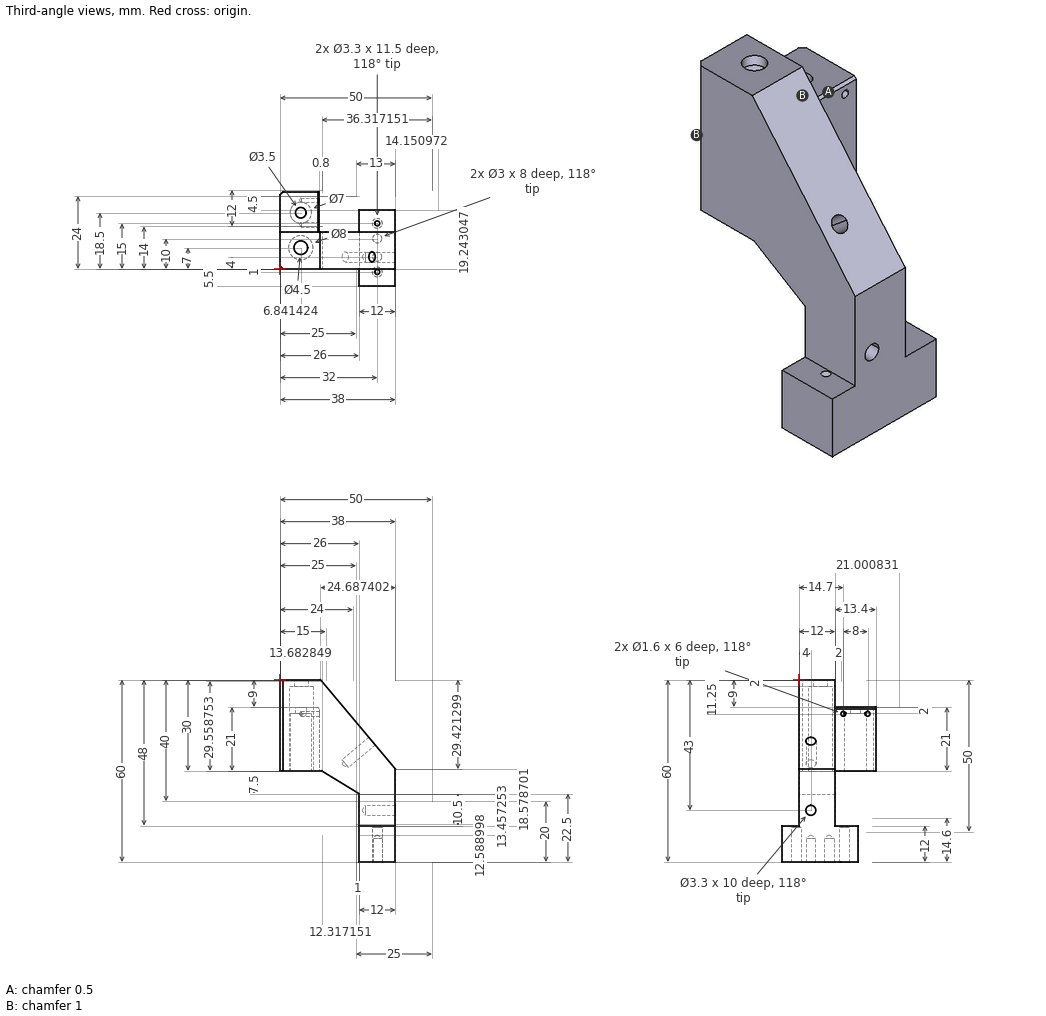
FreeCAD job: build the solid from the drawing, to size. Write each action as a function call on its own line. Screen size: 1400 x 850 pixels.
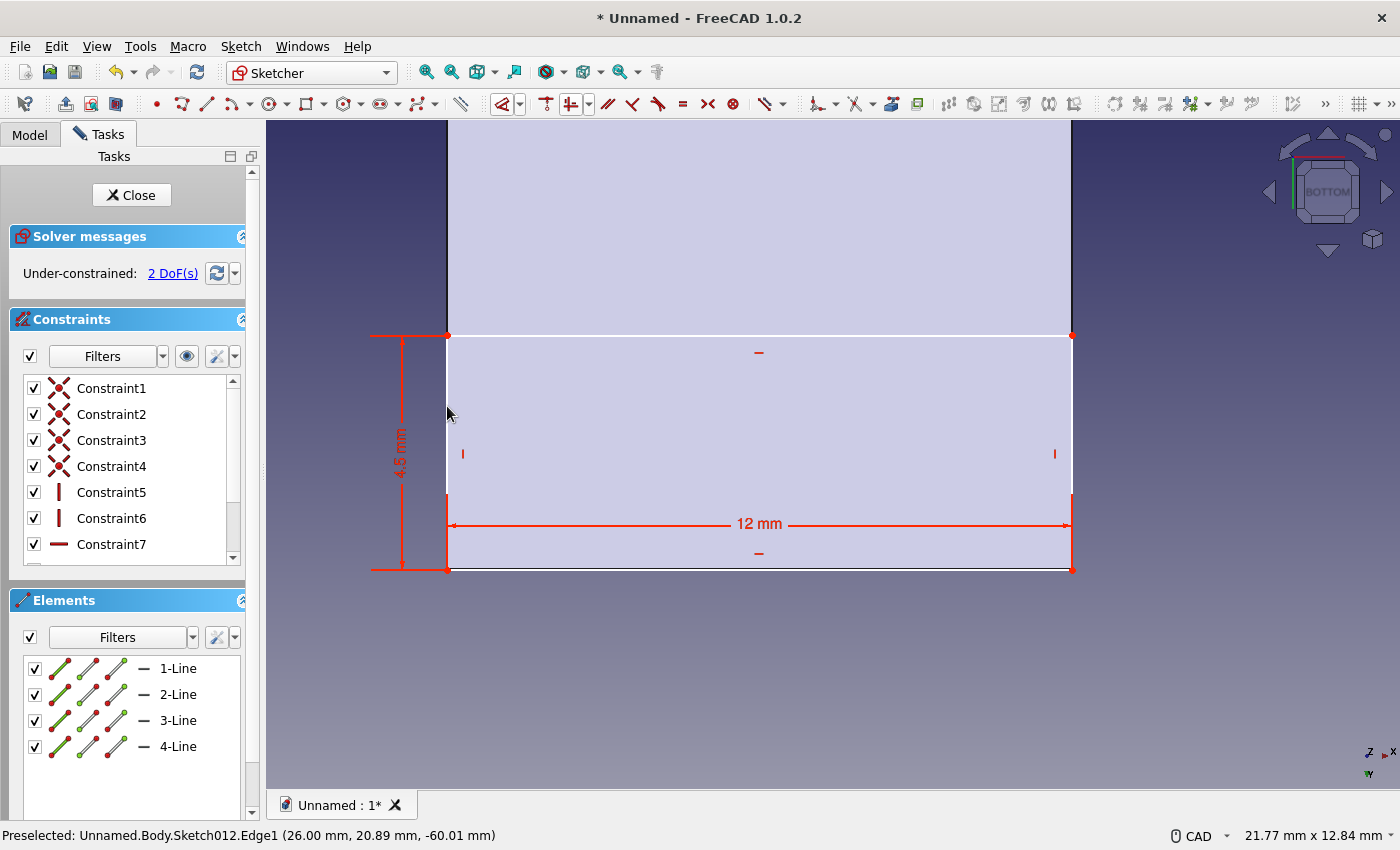
click(447, 336)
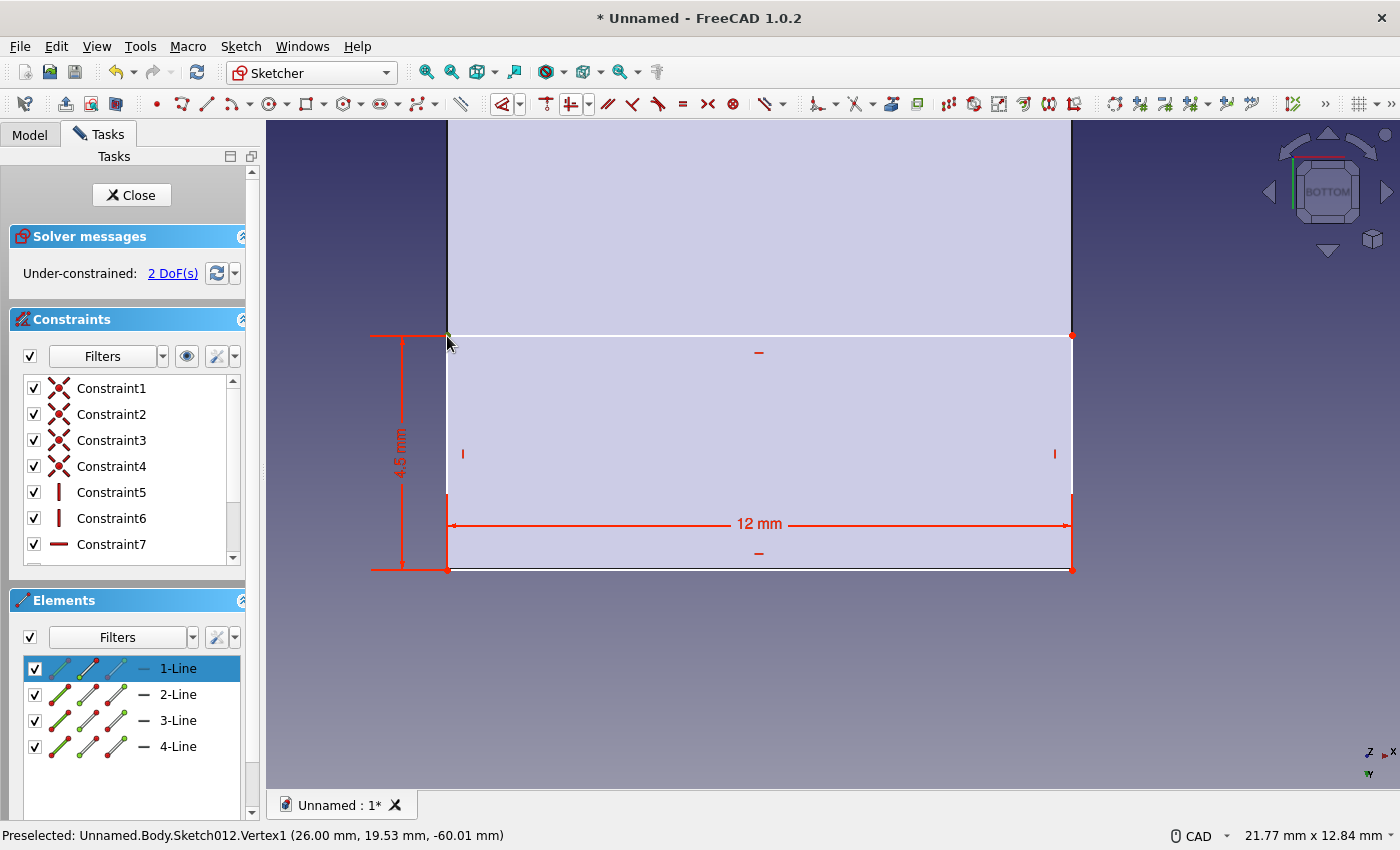
key(l)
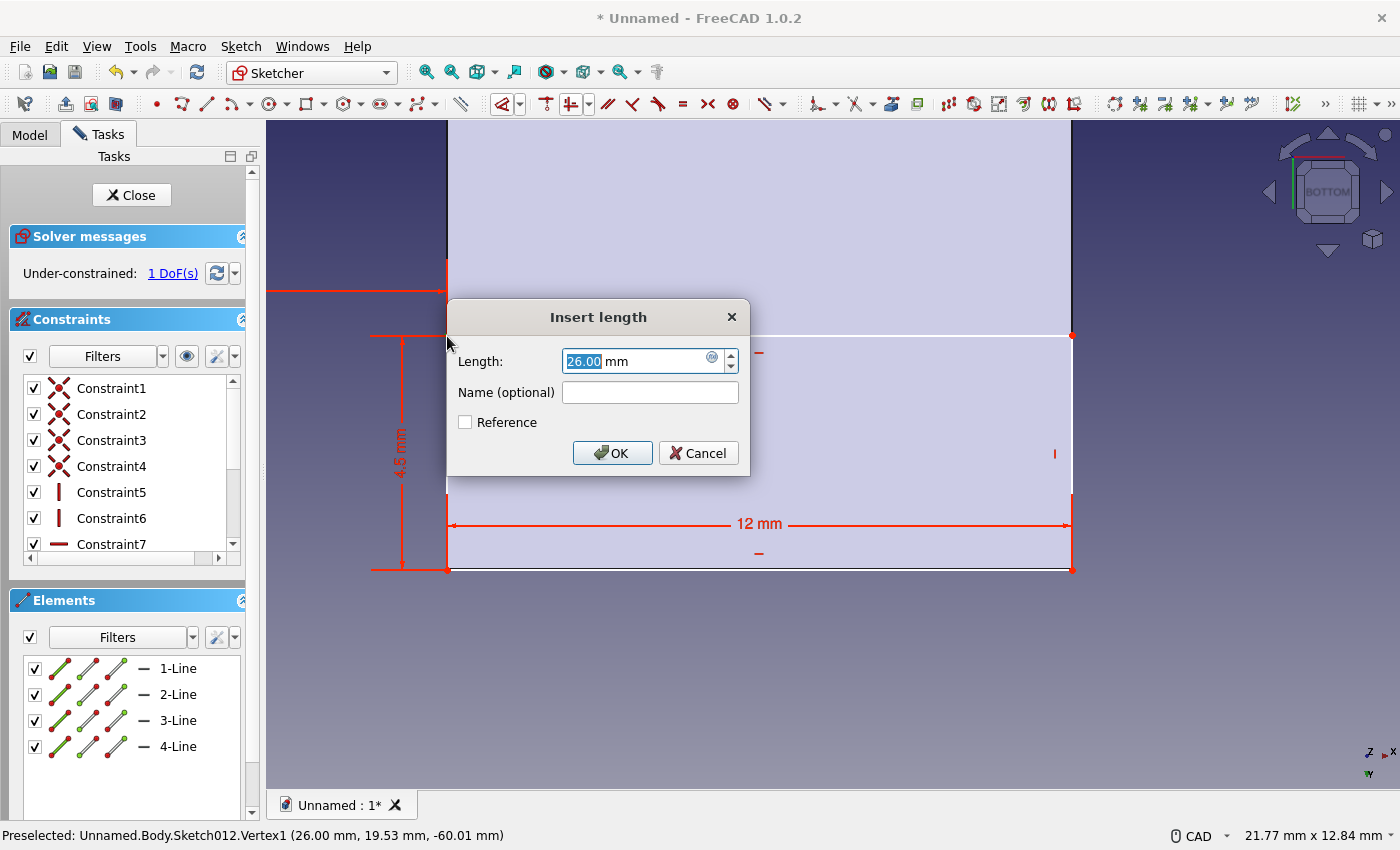
text(26)
key(Return)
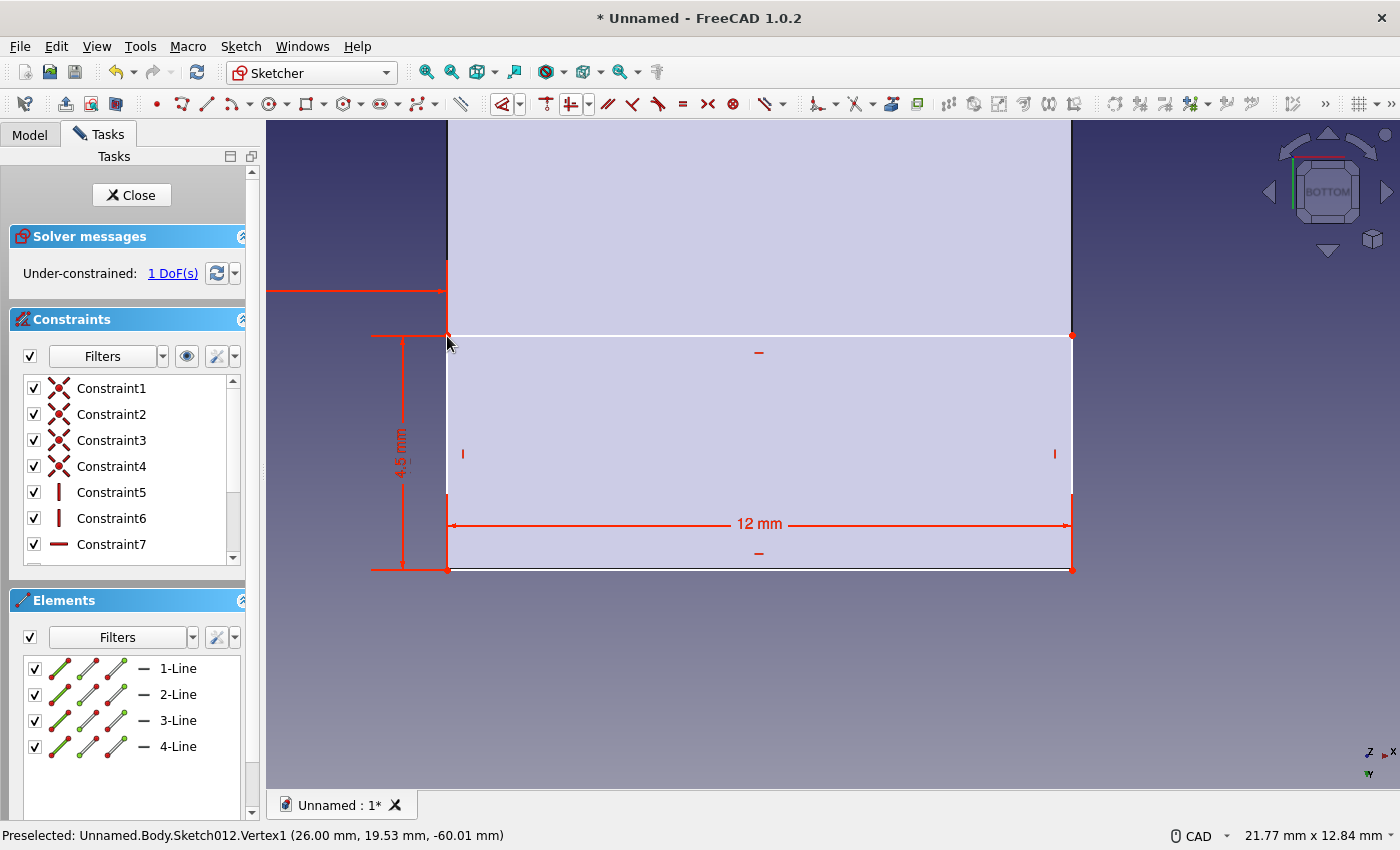
click(447, 570)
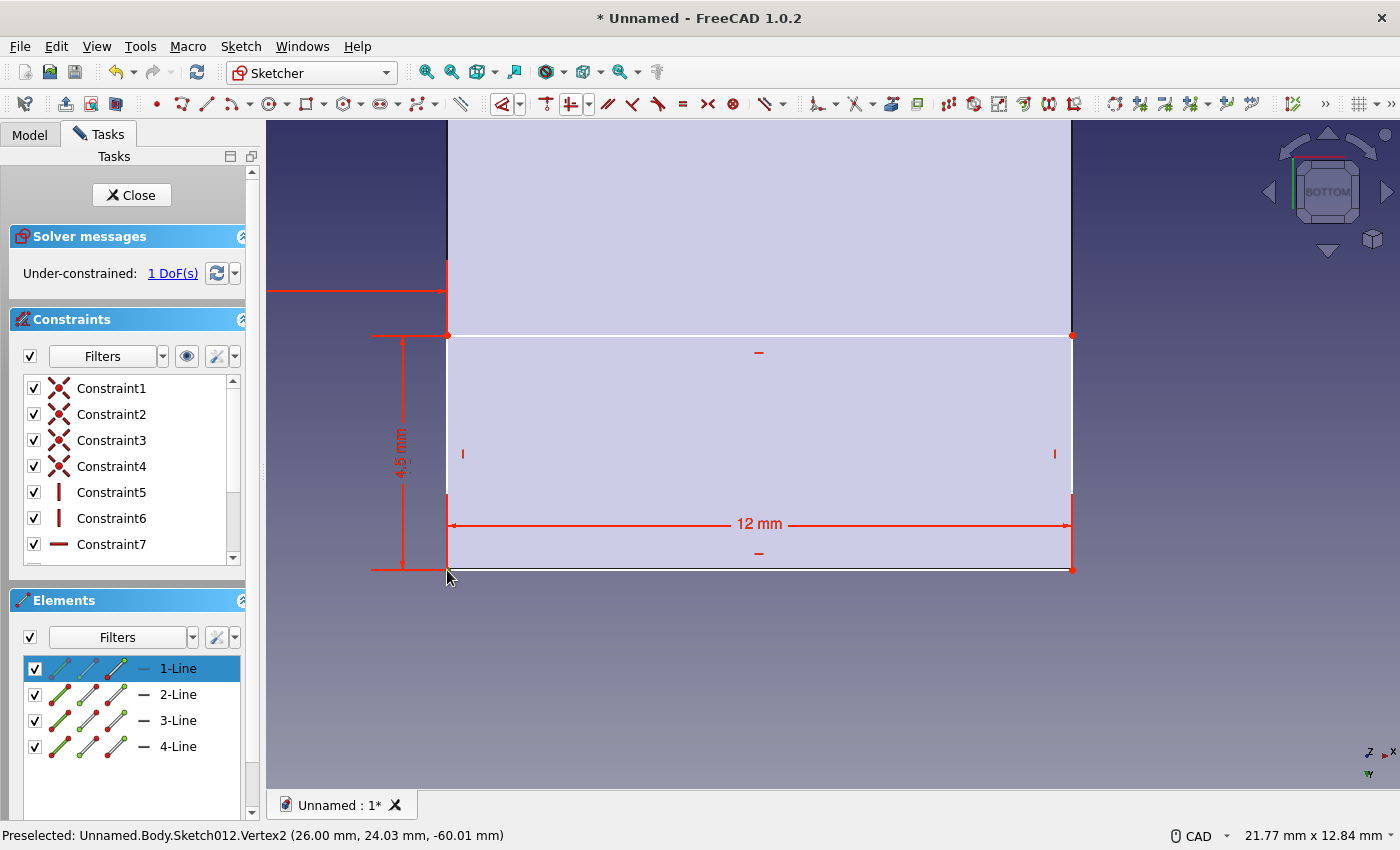
key(i)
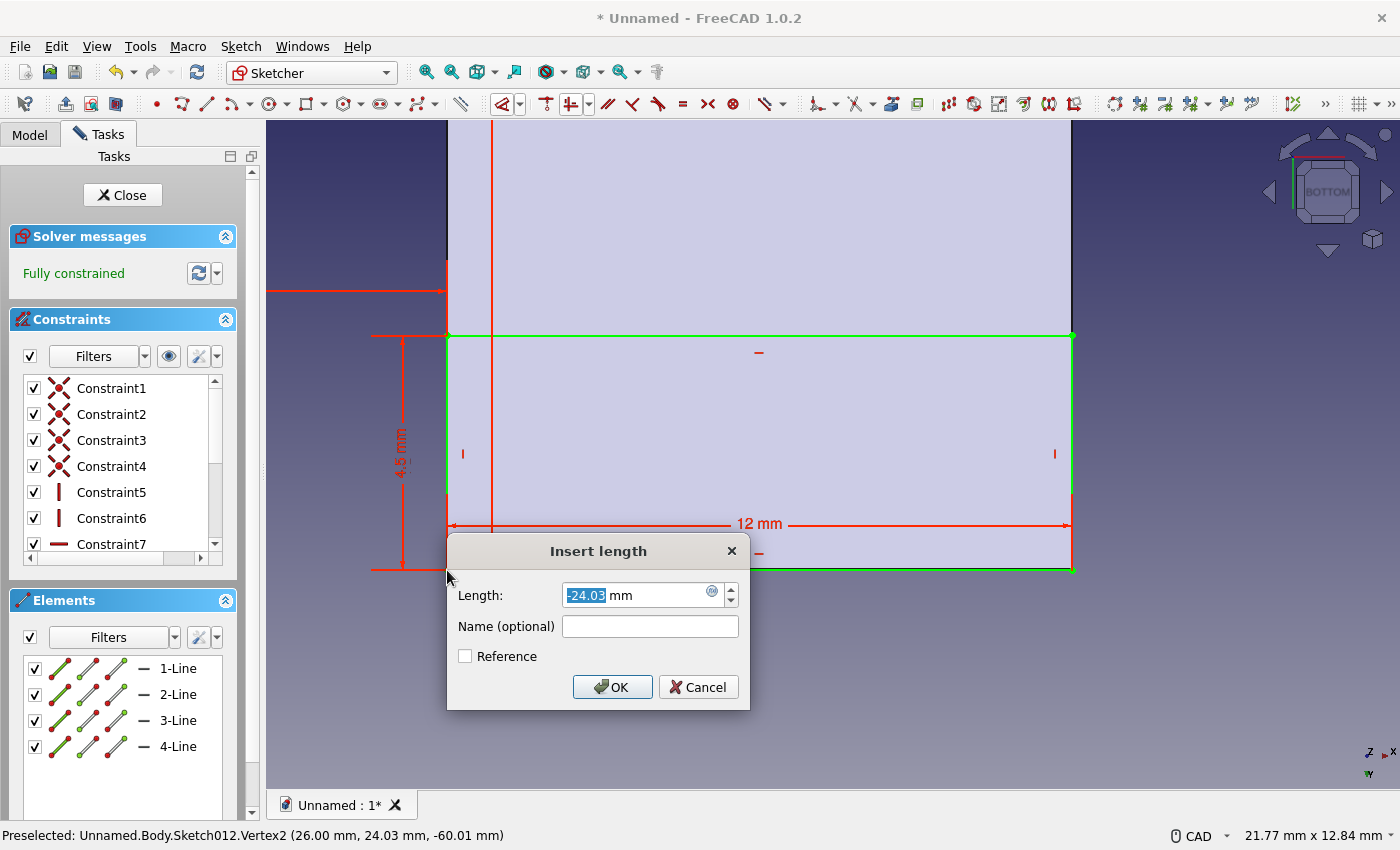
text(-24)
key(Return)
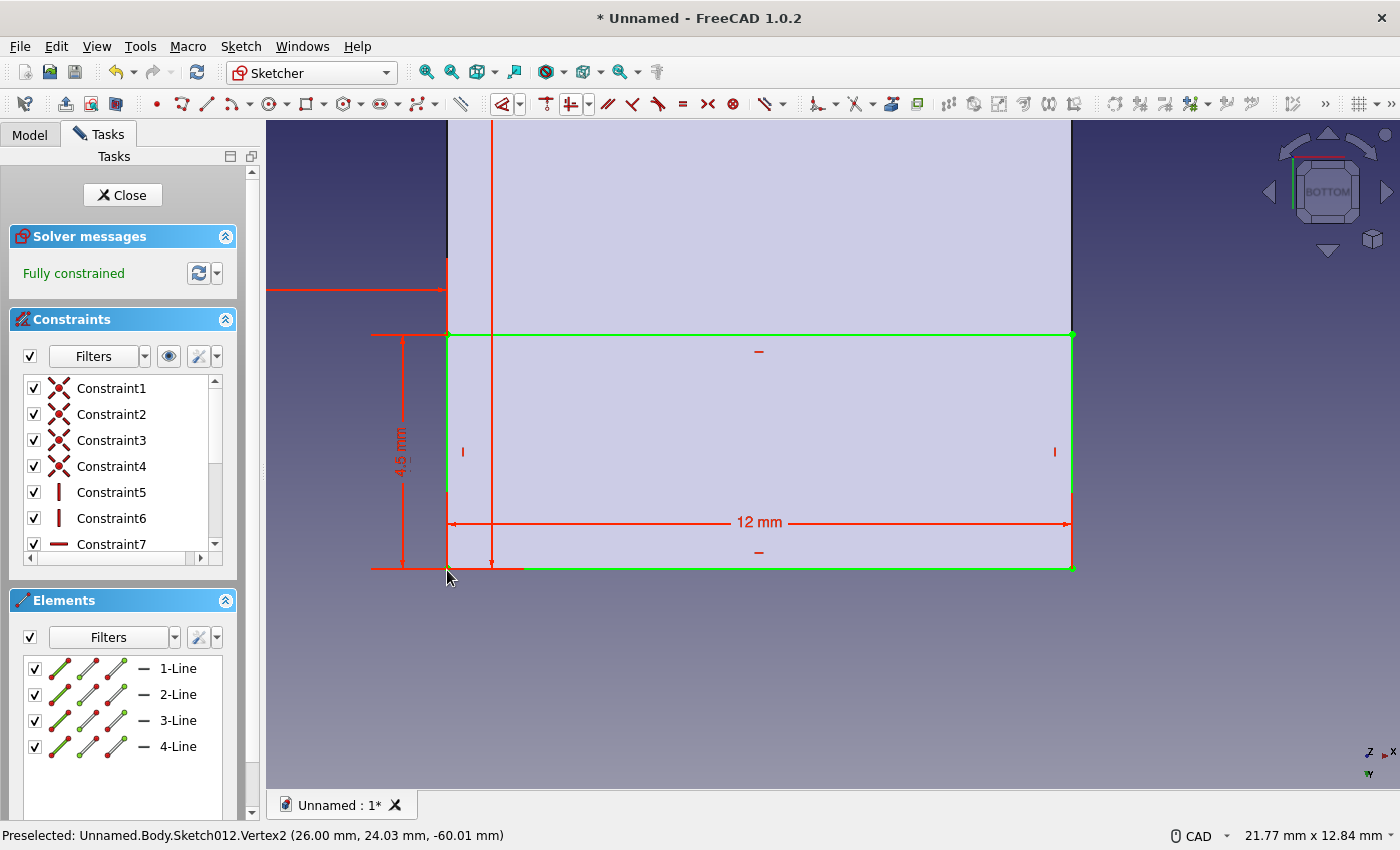
click(123, 195)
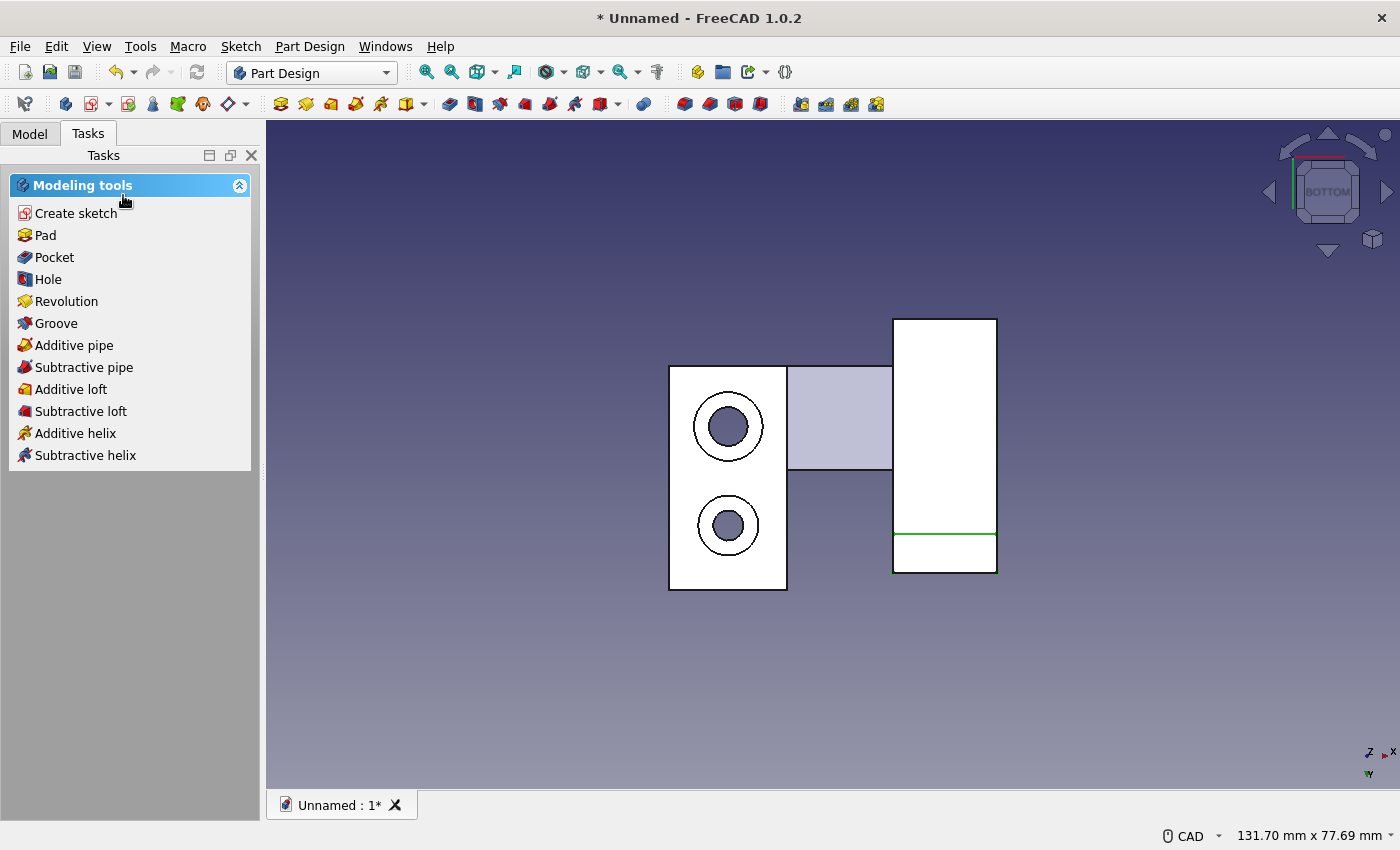
click(450, 104)